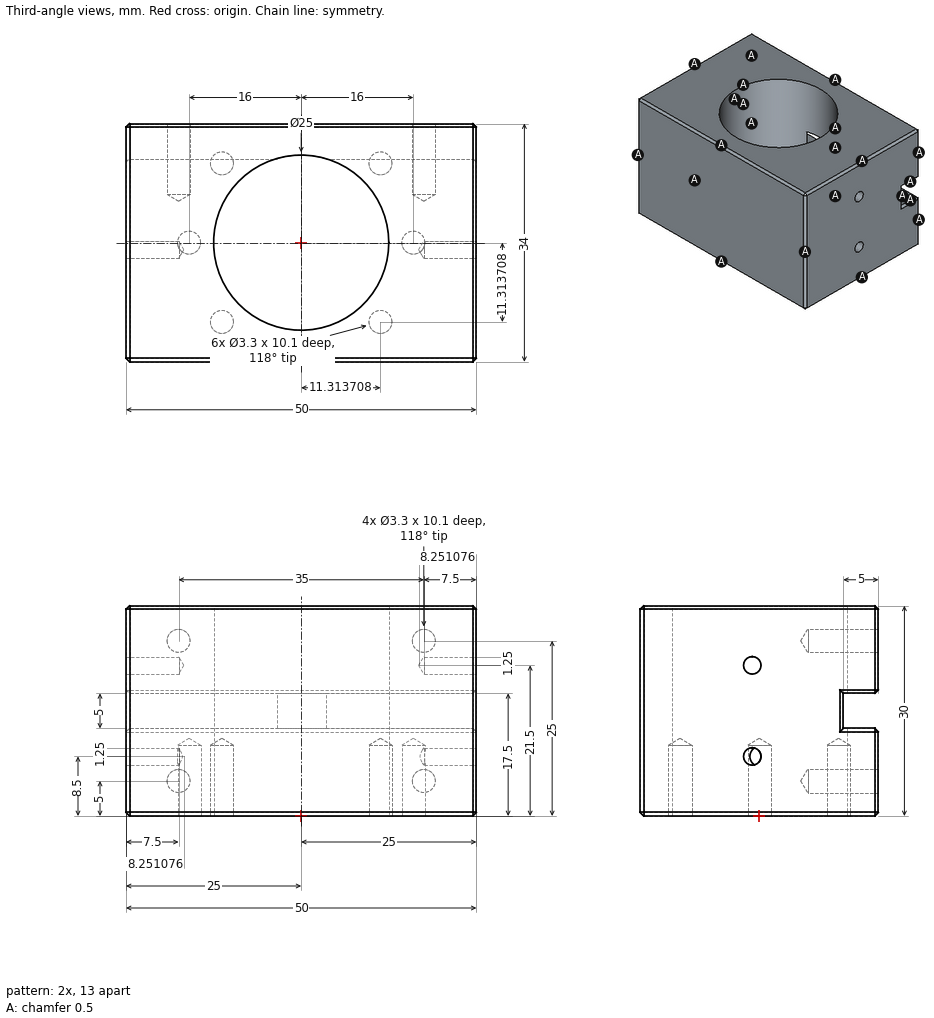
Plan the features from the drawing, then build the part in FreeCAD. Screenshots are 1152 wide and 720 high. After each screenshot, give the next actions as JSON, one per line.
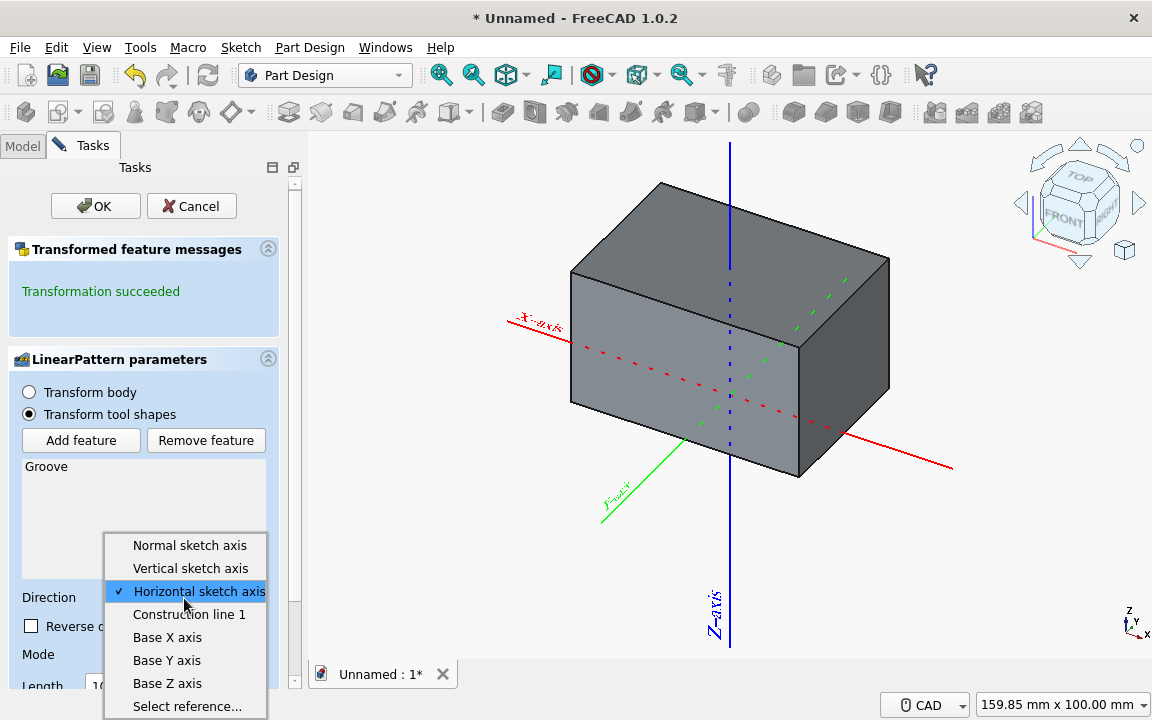
{"action": "left_click", "coordinate": [184, 684]}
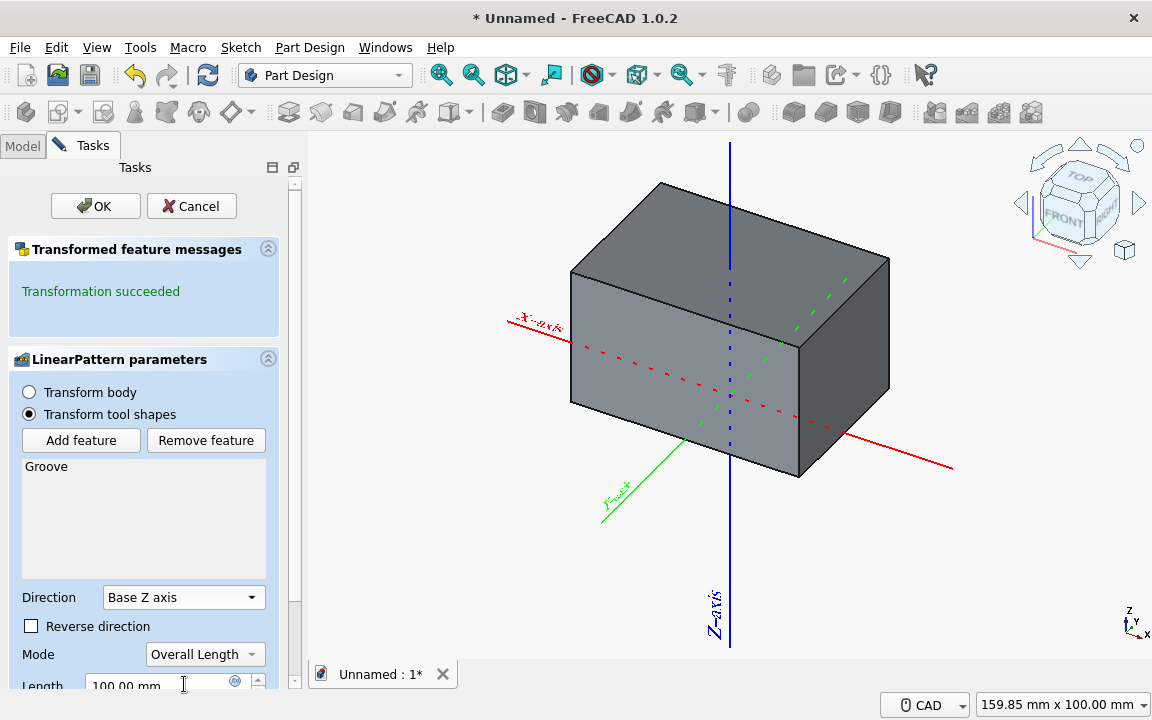
{"action": "left_click", "coordinate": [206, 654]}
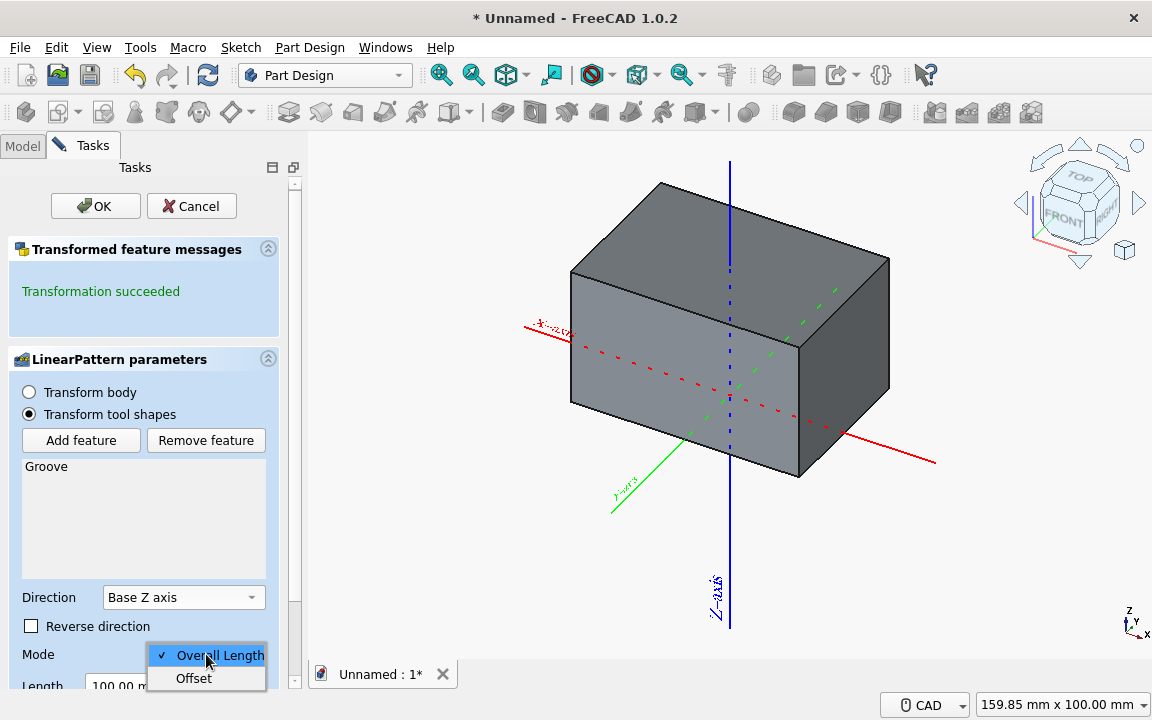
{"action": "left_click", "coordinate": [206, 678]}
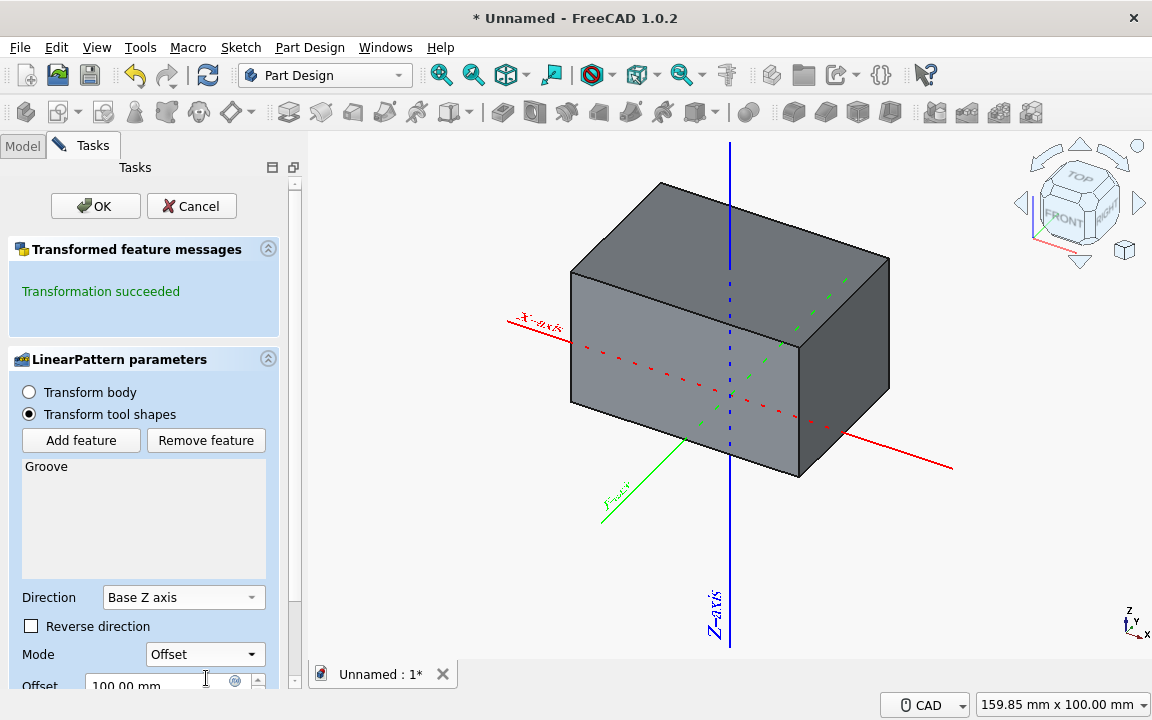
{"action": "scroll", "coordinate": [295, 432], "scroll_direction": "down", "scroll_amount": 2}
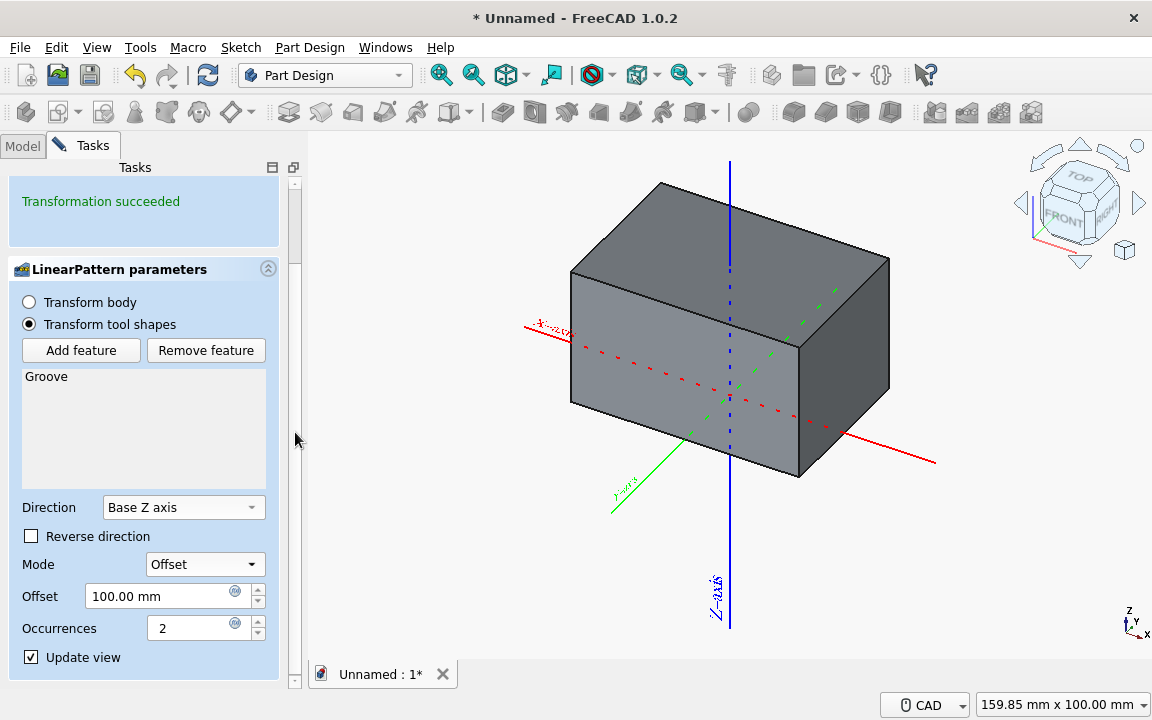
{"action": "triple_click", "coordinate": [168, 596]}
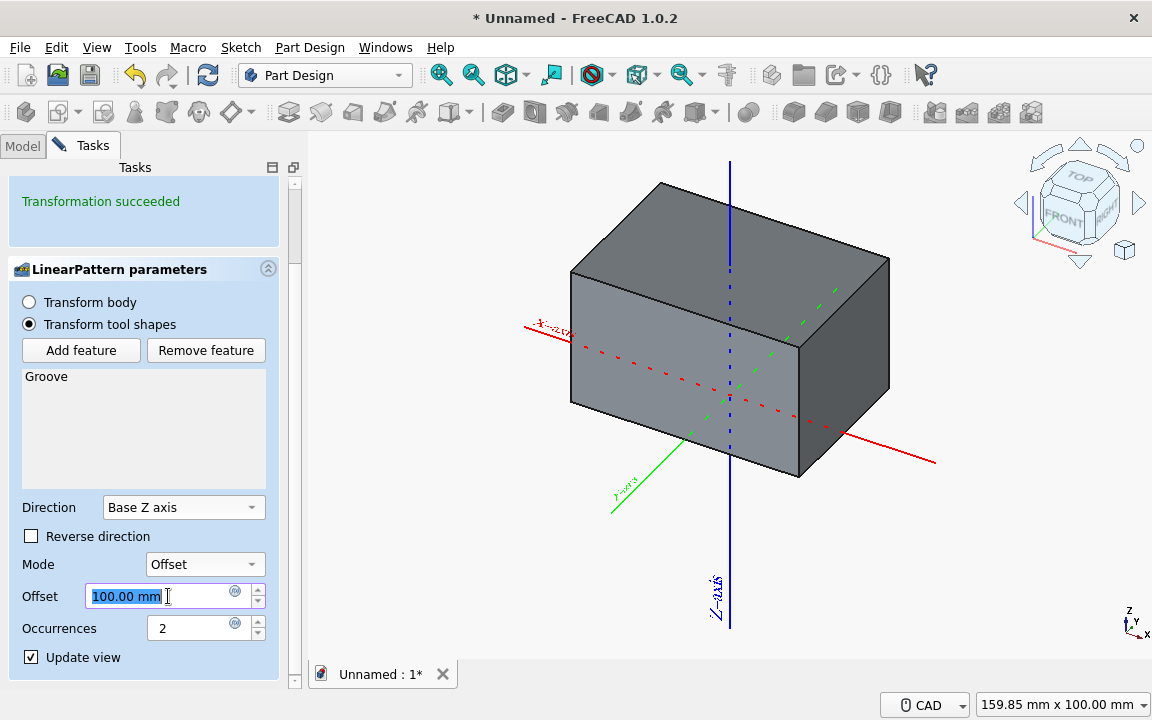
{"action": "type", "text": "13"}
{"action": "key", "text": "Tab"}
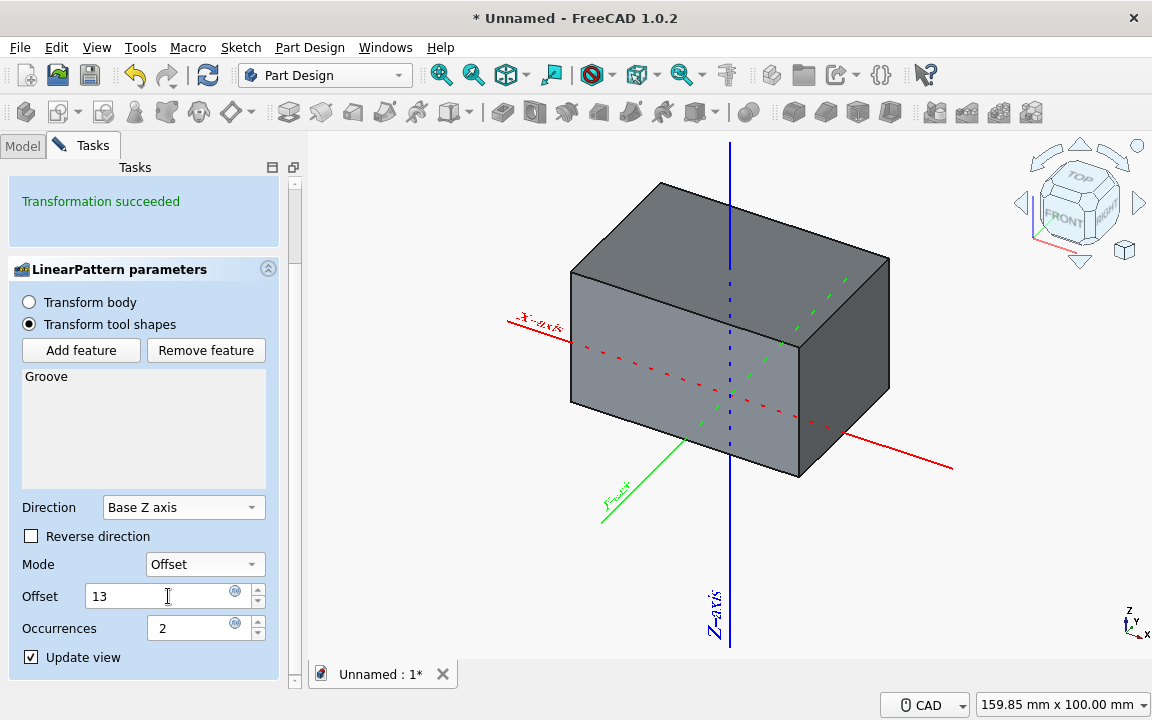
{"action": "triple_click", "coordinate": [198, 628]}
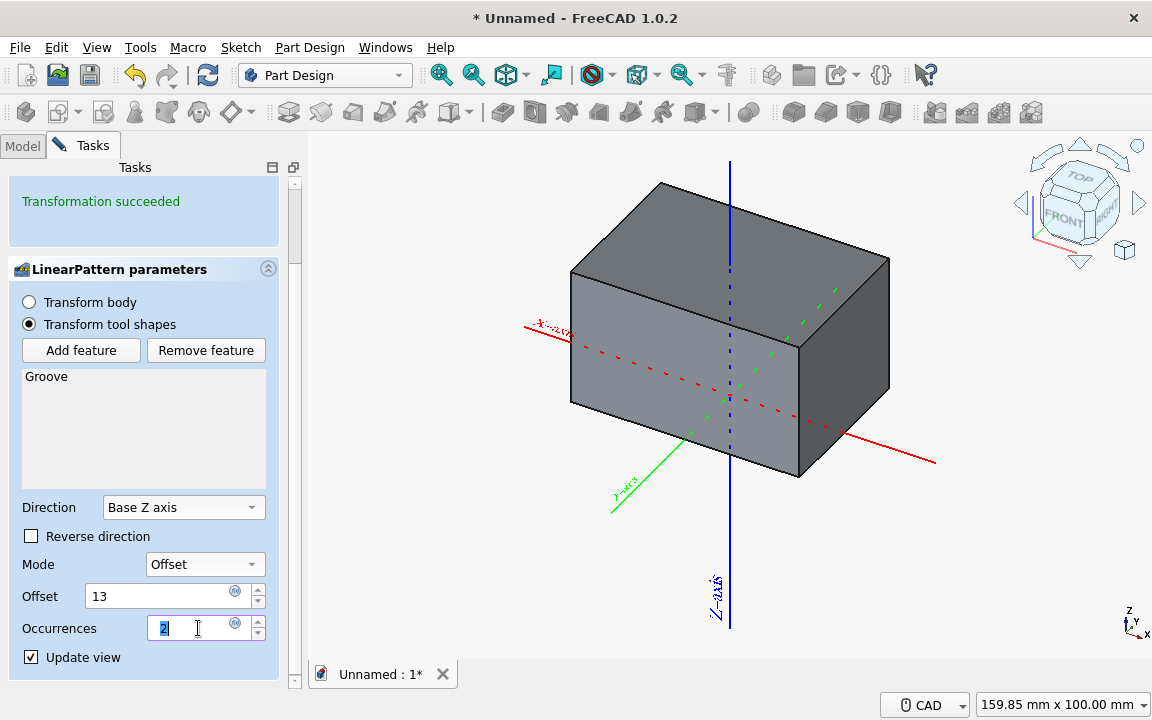
{"action": "type", "text": "2"}
{"action": "key", "text": "Tab"}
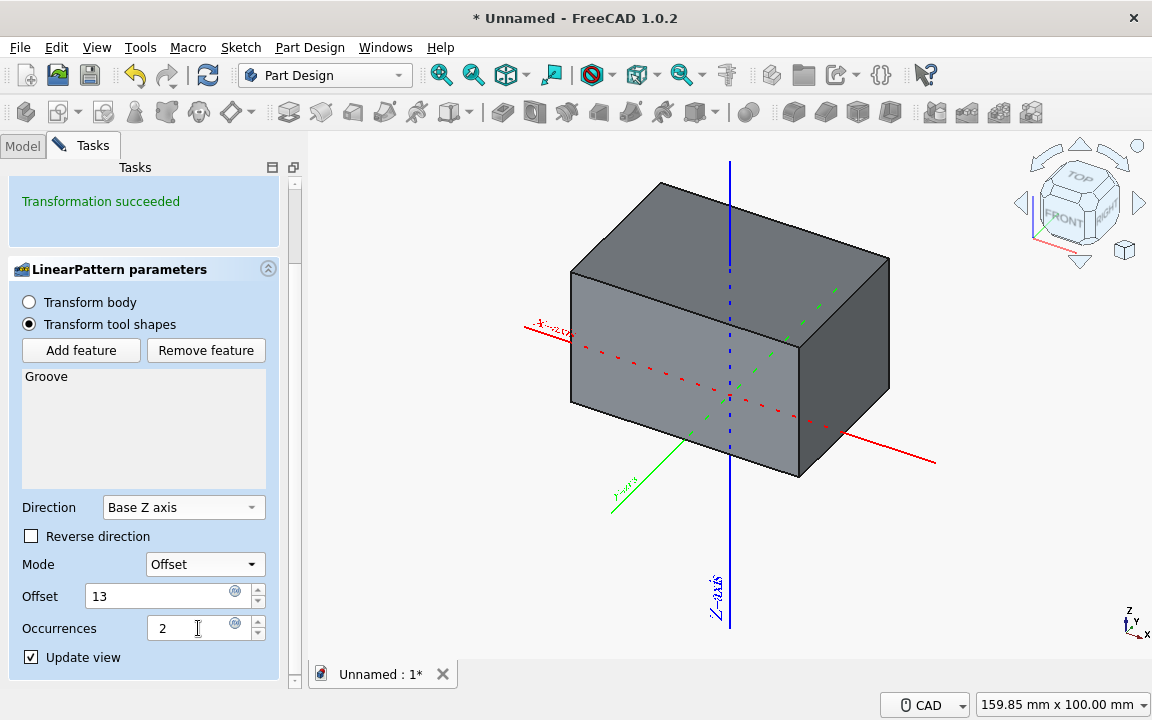
{"action": "scroll", "coordinate": [295, 432], "scroll_direction": "up", "scroll_amount": 3}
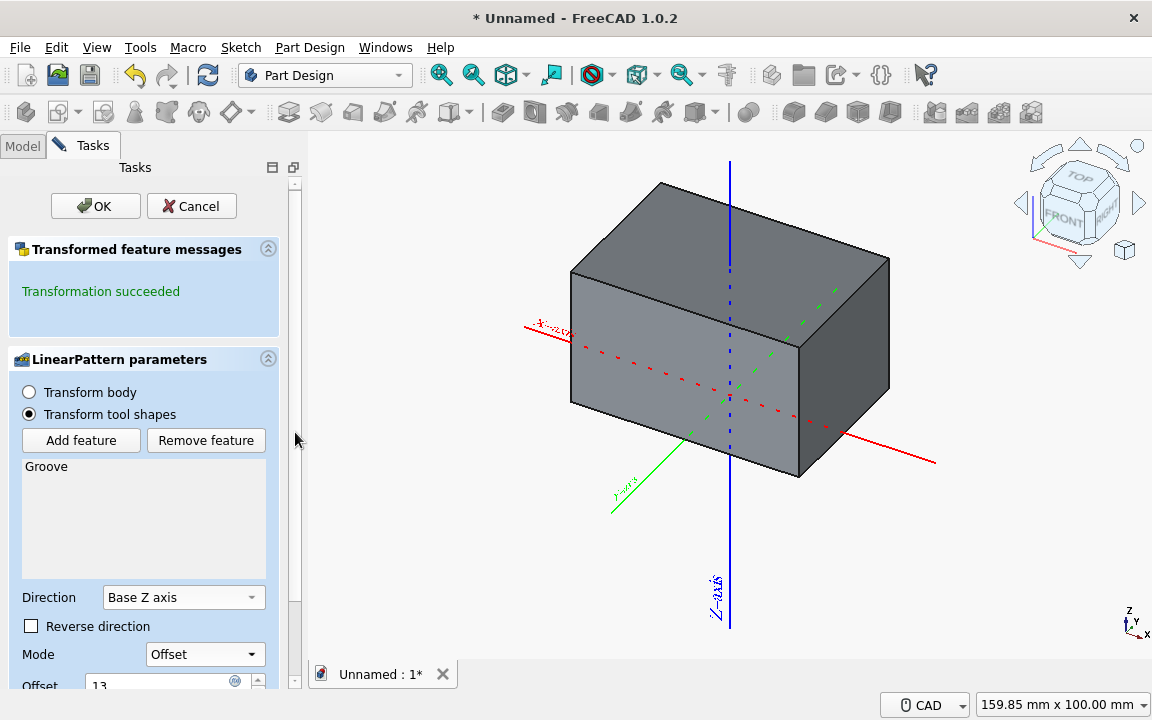
{"action": "left_click", "coordinate": [96, 206]}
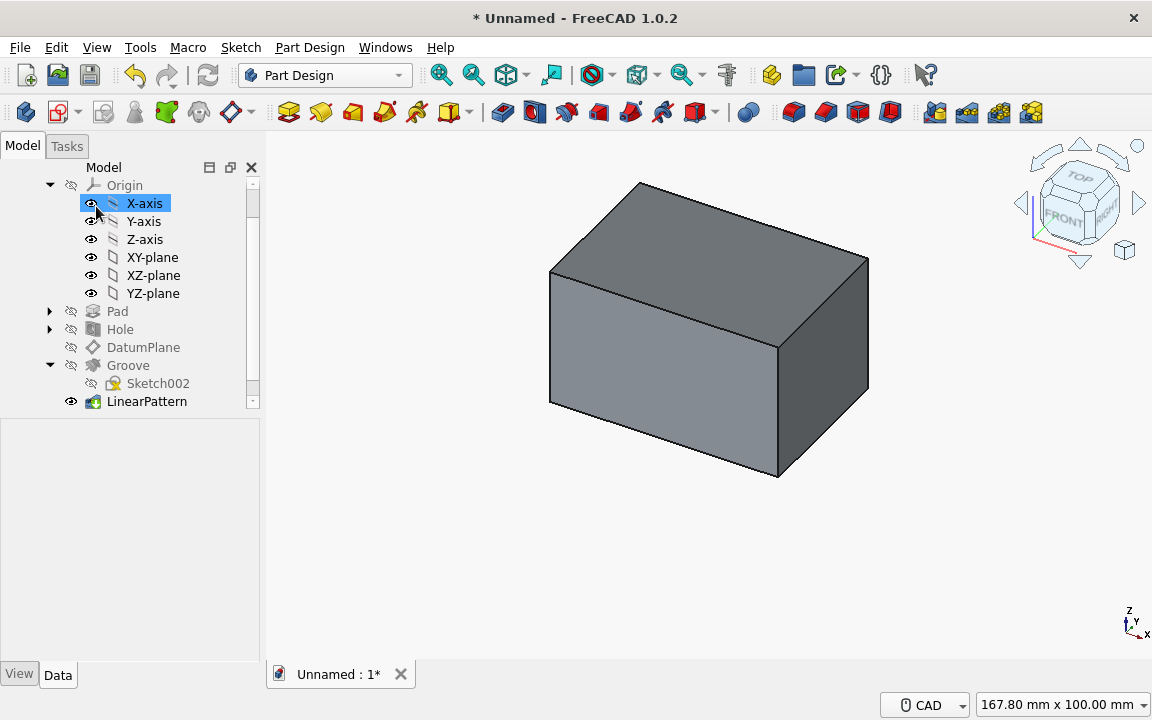
{"action": "left_click", "coordinate": [116, 365]}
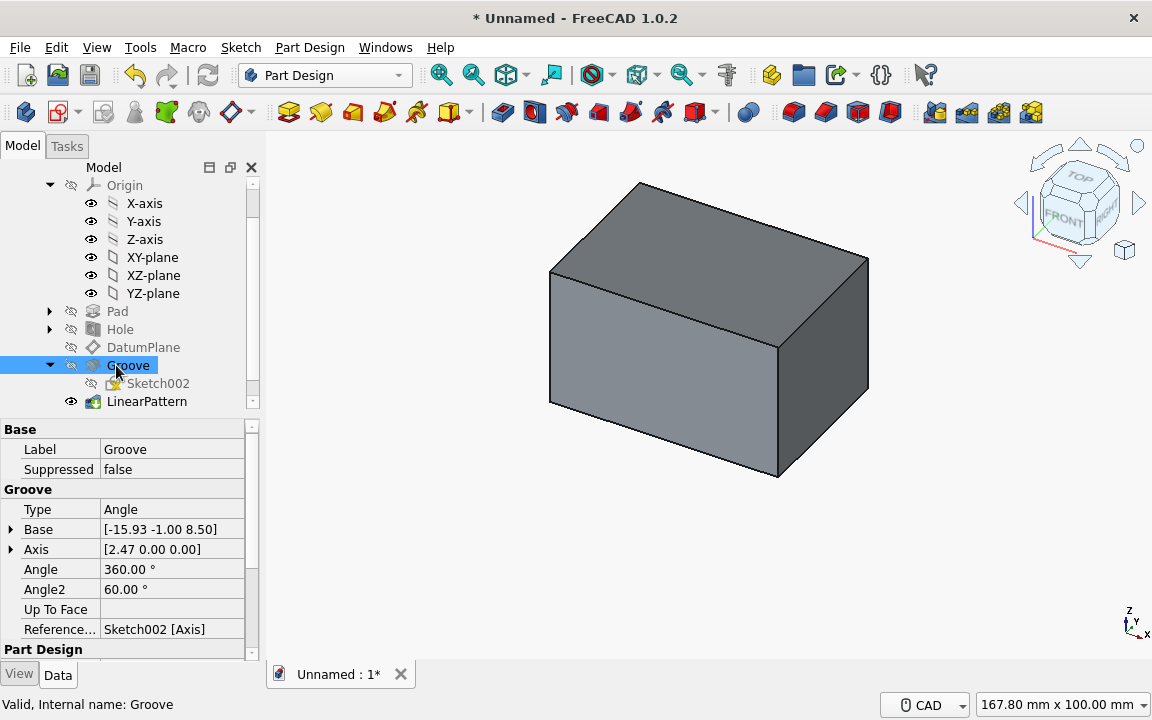
{"action": "left_click", "coordinate": [936, 112]}